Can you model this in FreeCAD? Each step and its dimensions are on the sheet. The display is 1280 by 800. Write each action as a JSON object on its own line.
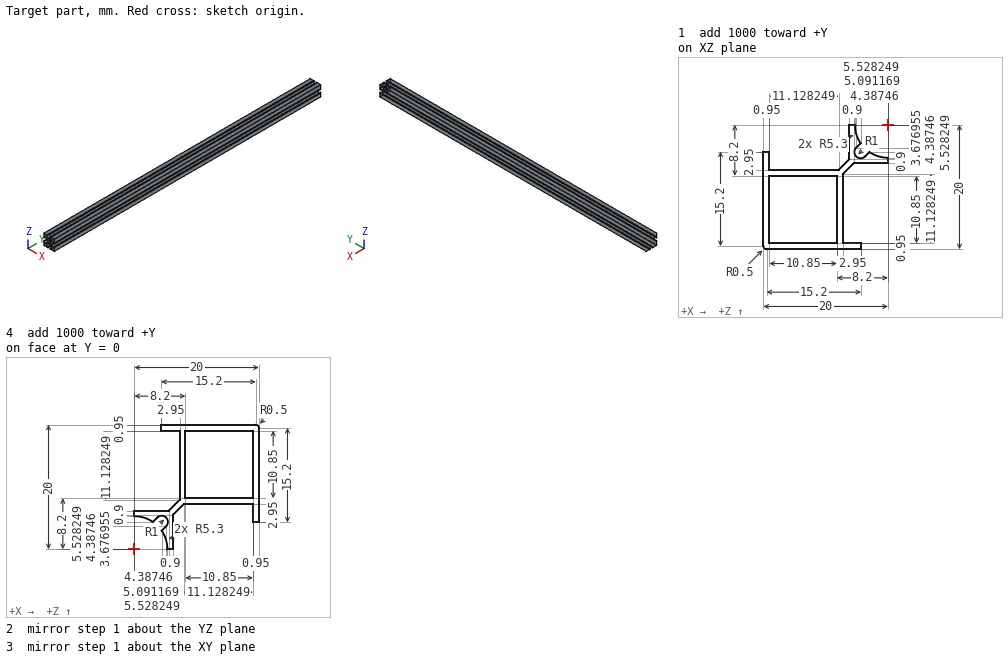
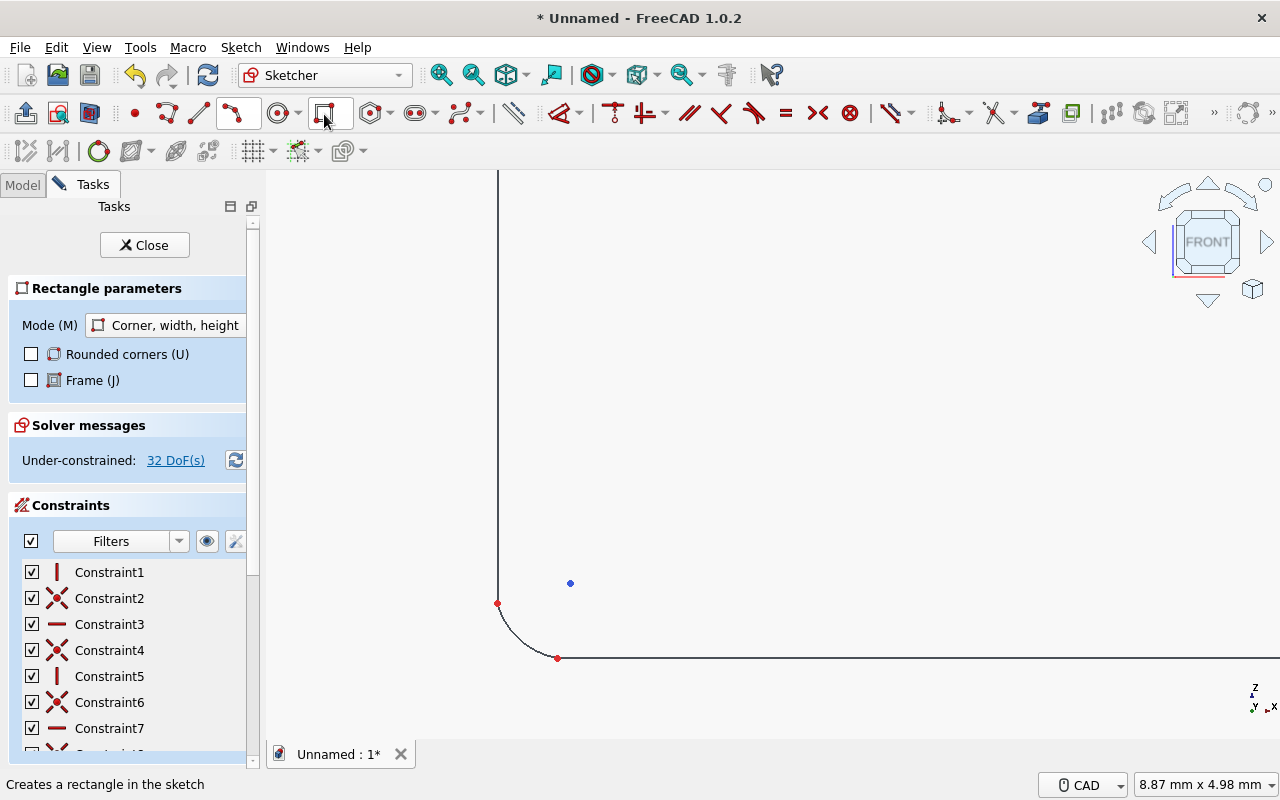
{"action": "scroll", "coordinate": [519, 642], "scroll_direction": "down", "scroll_amount": 9}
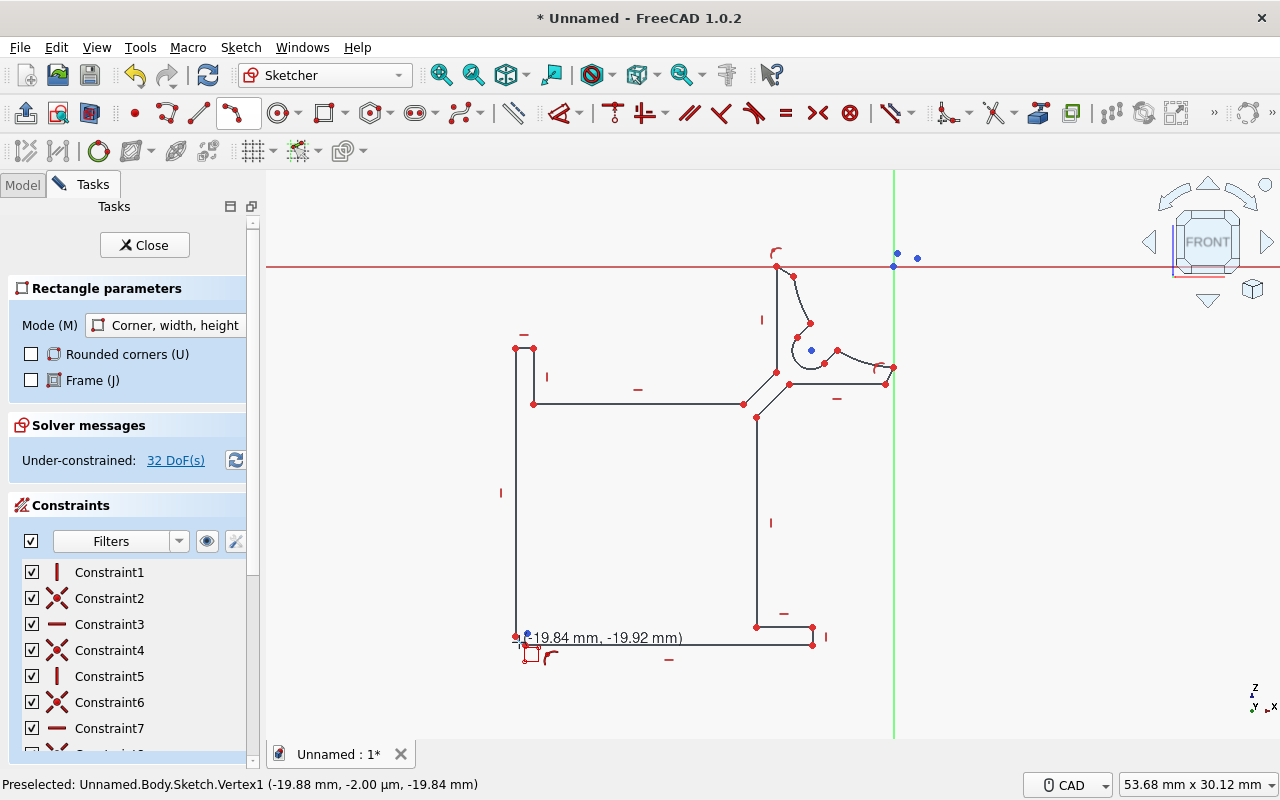
{"action": "left_click", "coordinate": [534, 422]}
{"action": "mouse_move", "coordinate": [739, 626]}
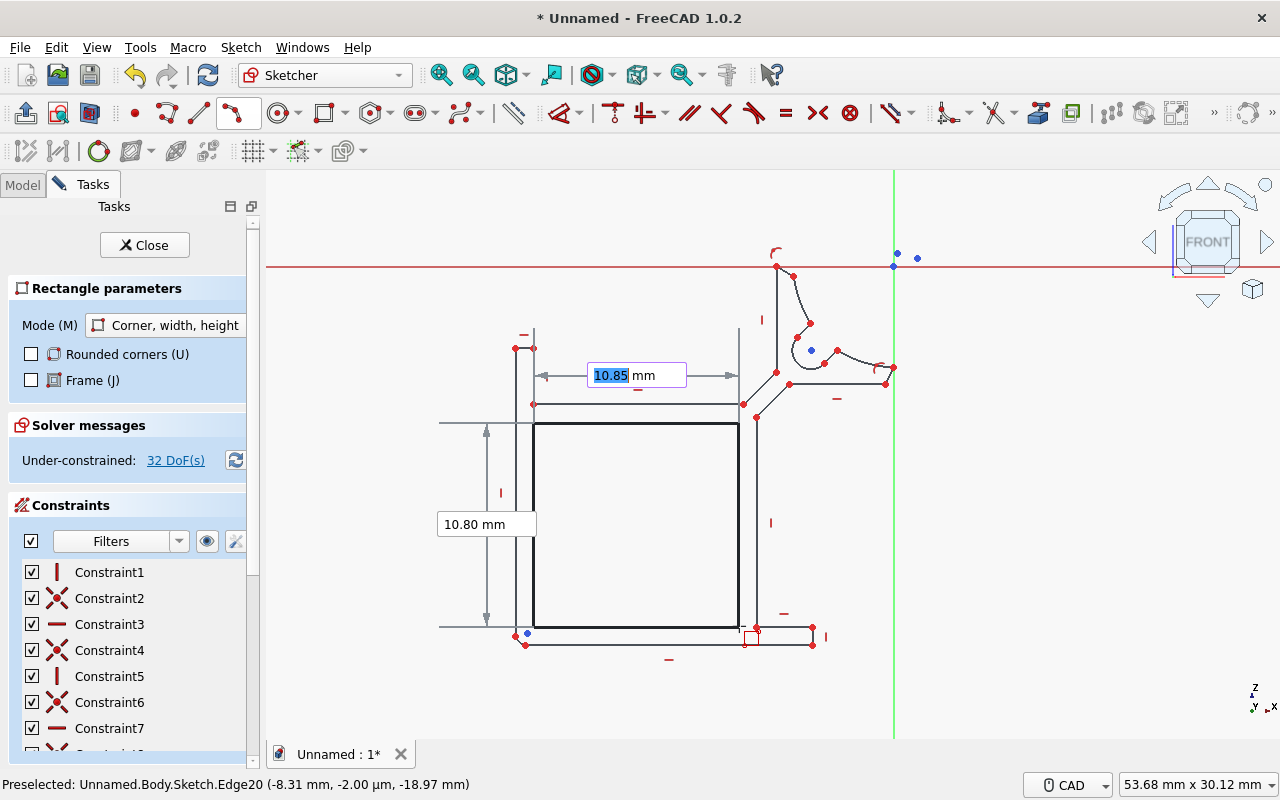
{"action": "type", "text": "10.85"}
{"action": "key", "text": "Tab"}
{"action": "type", "text": "10.85"}
{"action": "key", "text": "Return"}
{"action": "key", "text": "Escape"}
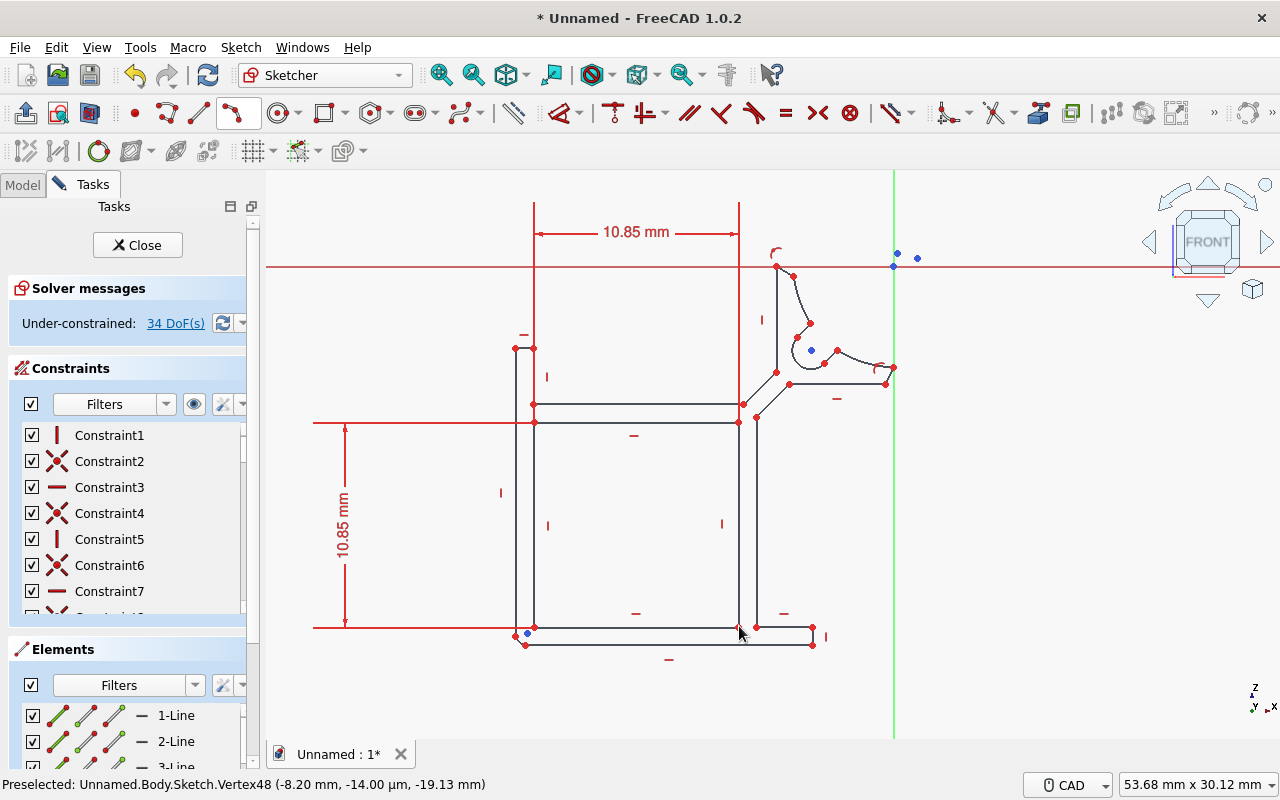
{"action": "left_click", "coordinate": [516, 550]}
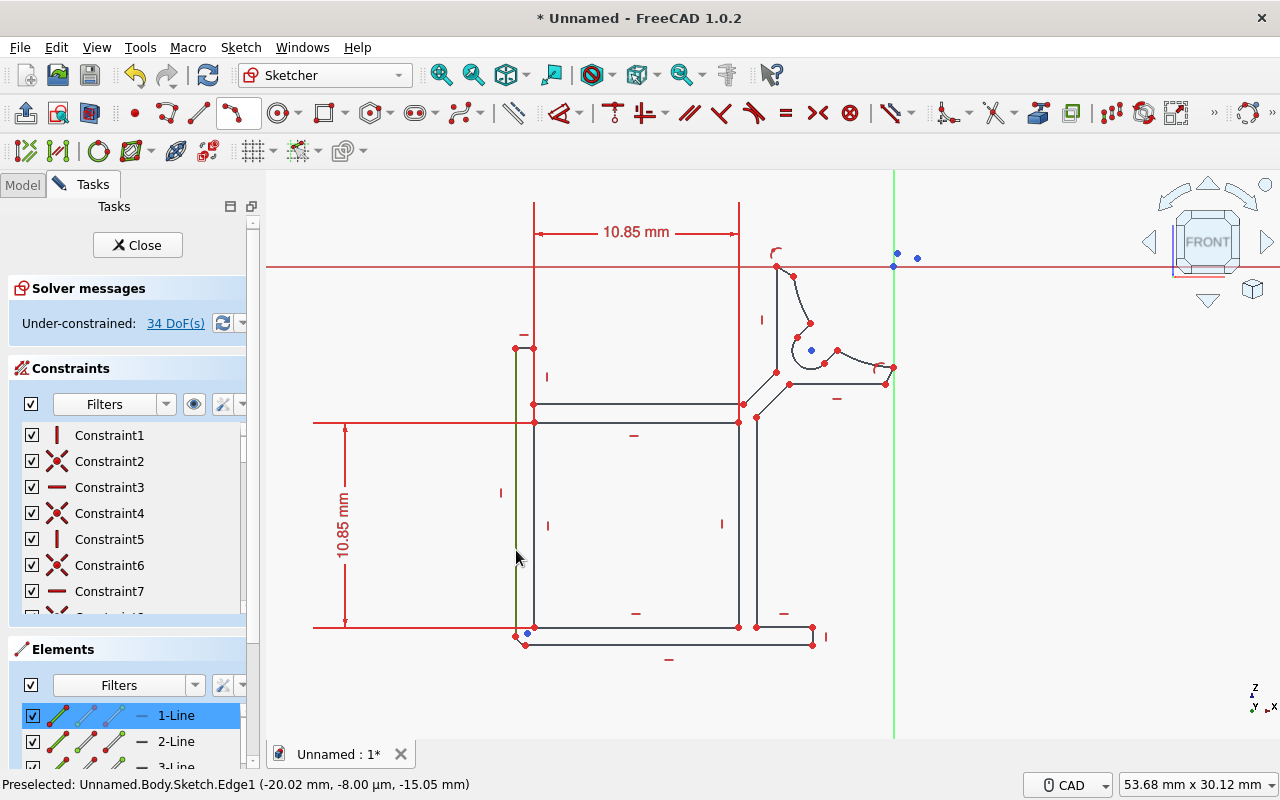
{"action": "scroll", "coordinate": [519, 642], "scroll_direction": "up", "scroll_amount": 4}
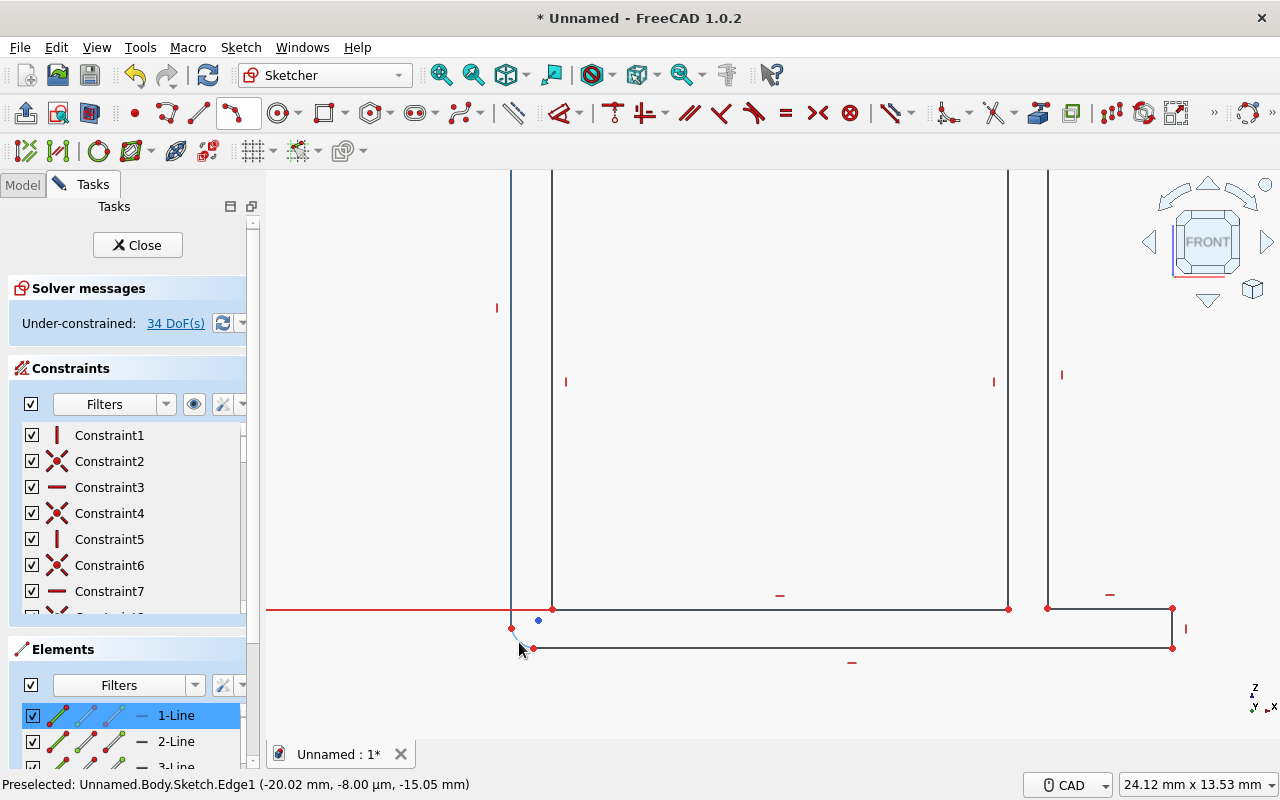
{"action": "left_click", "coordinate": [519, 642]}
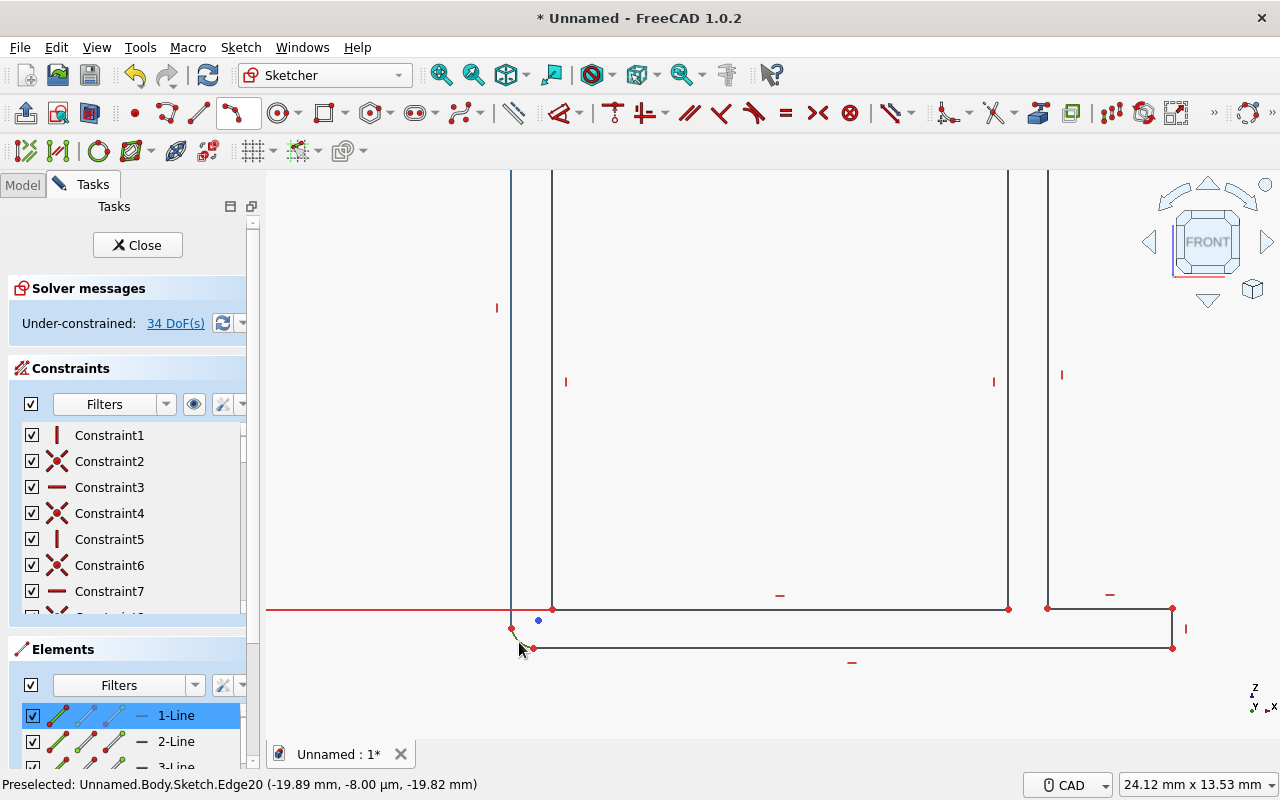
{"action": "left_click", "coordinate": [754, 114]}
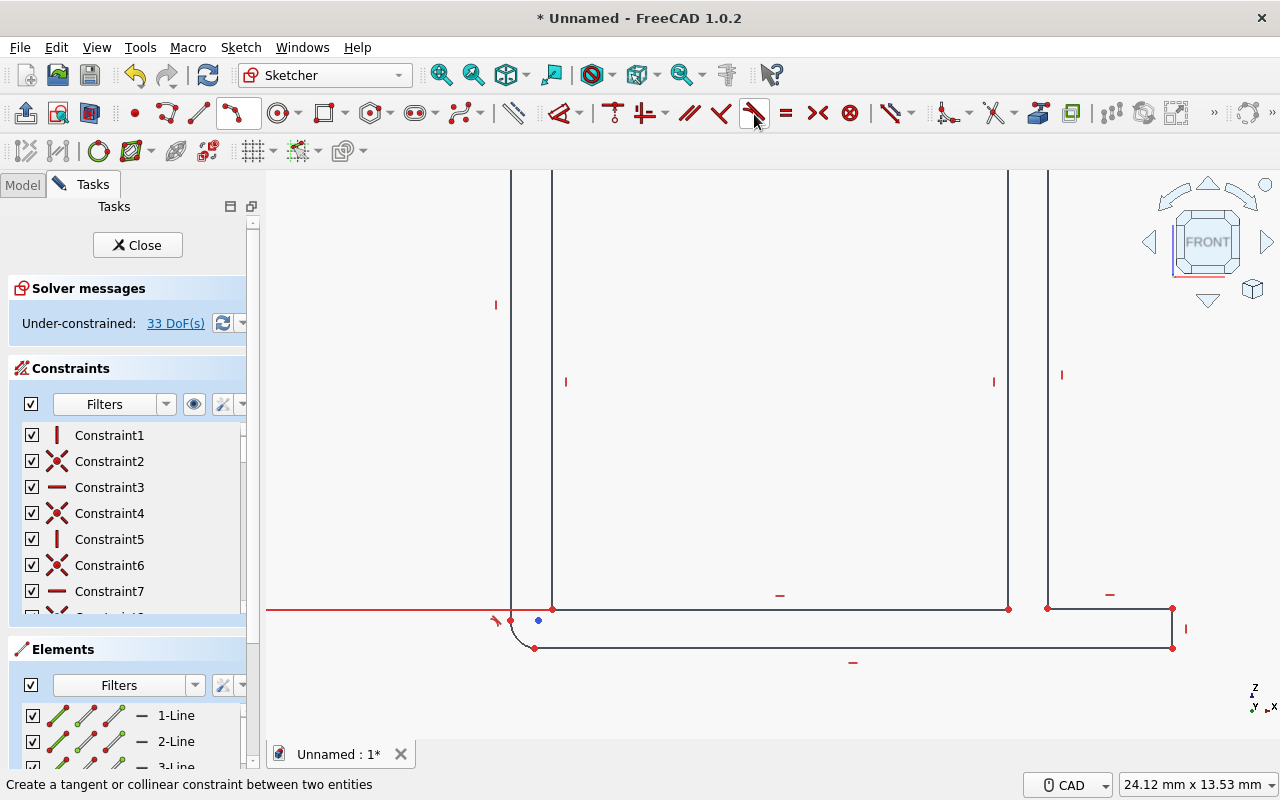
{"action": "scroll", "coordinate": [518, 641], "scroll_direction": "down", "scroll_amount": 4}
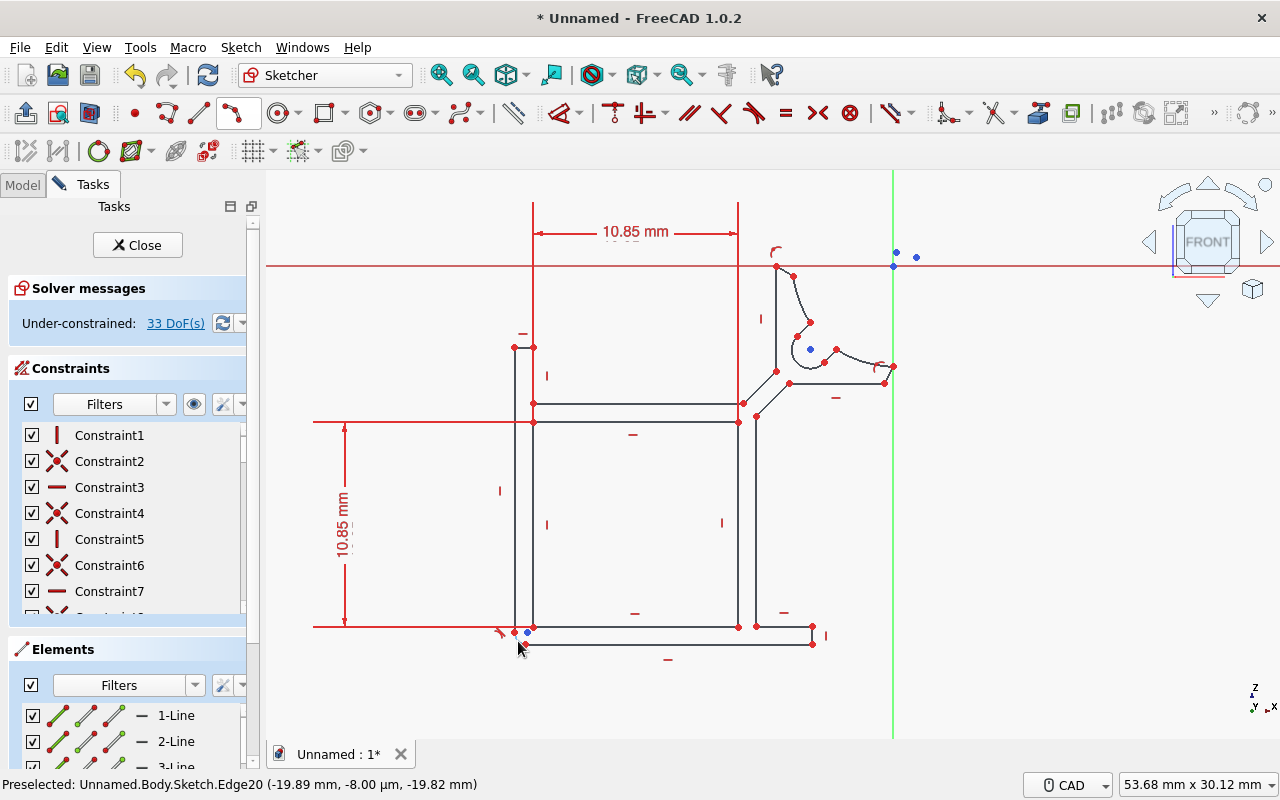
{"action": "scroll", "coordinate": [806, 327], "scroll_direction": "up", "scroll_amount": 5}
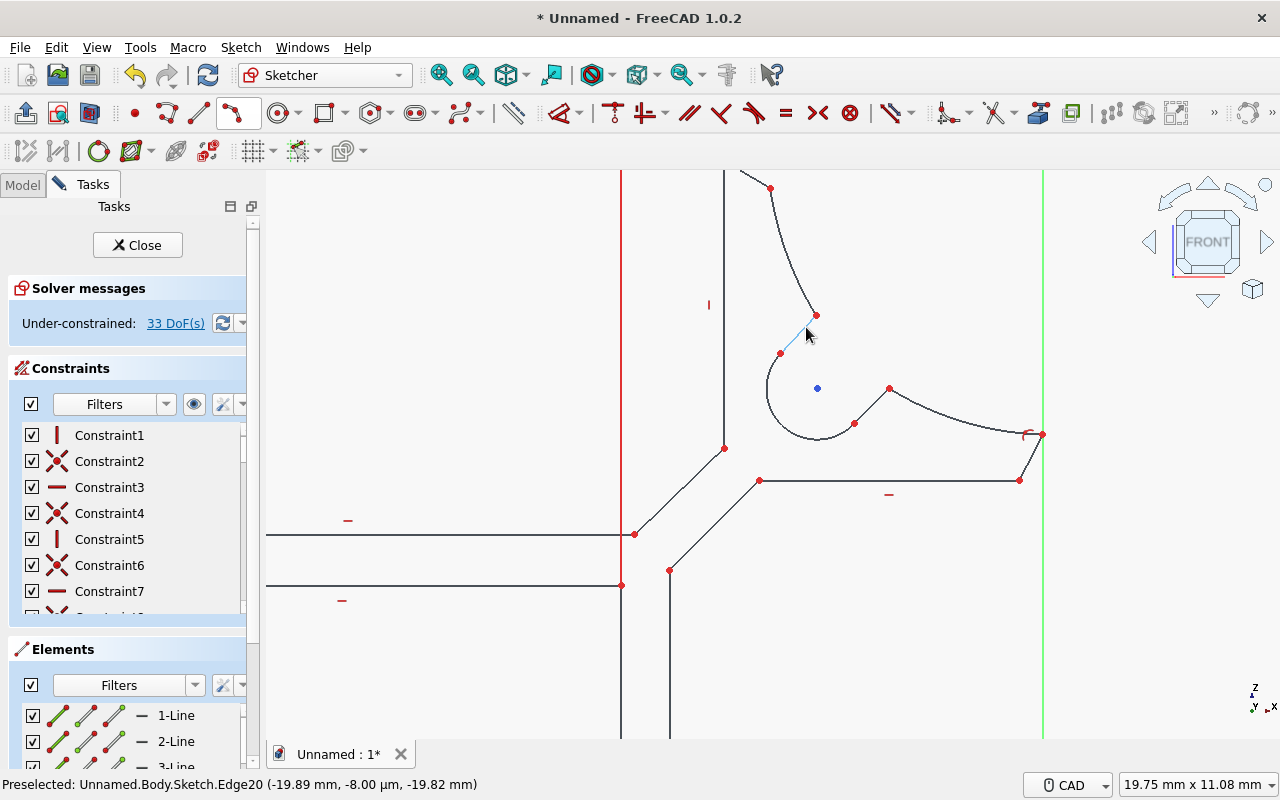
{"action": "left_click", "coordinate": [806, 327]}